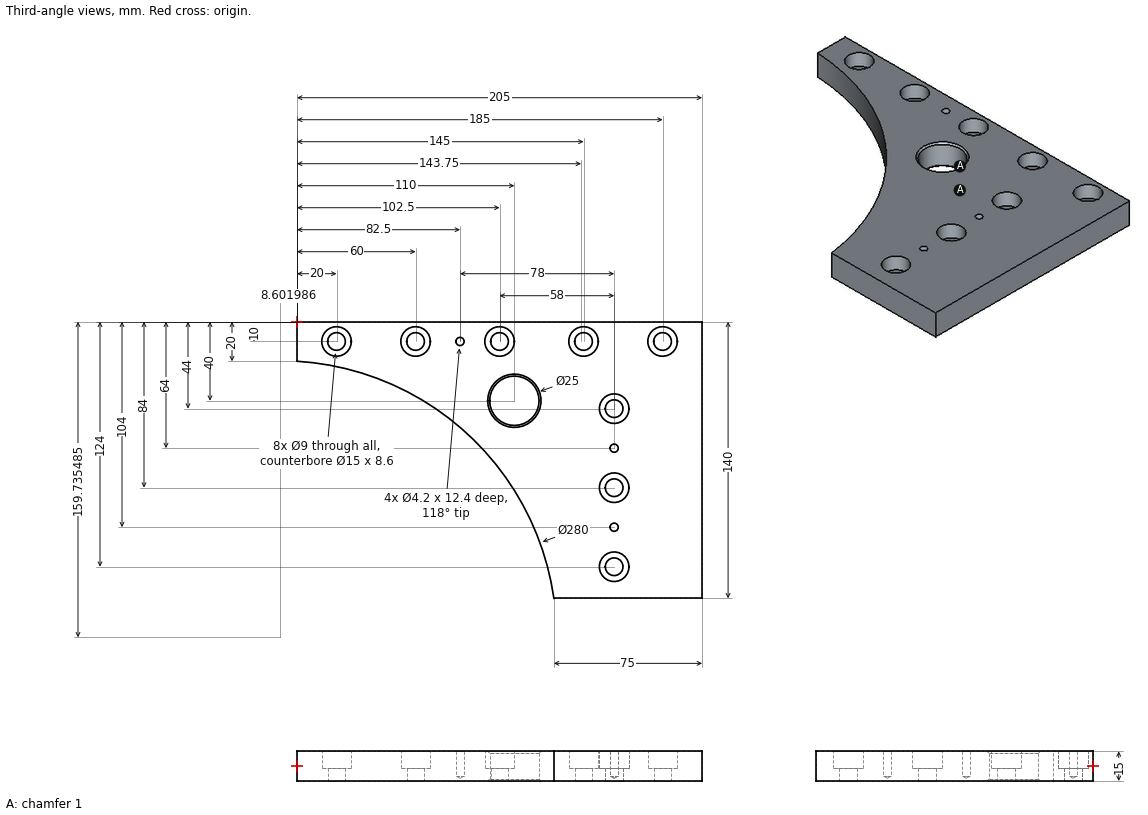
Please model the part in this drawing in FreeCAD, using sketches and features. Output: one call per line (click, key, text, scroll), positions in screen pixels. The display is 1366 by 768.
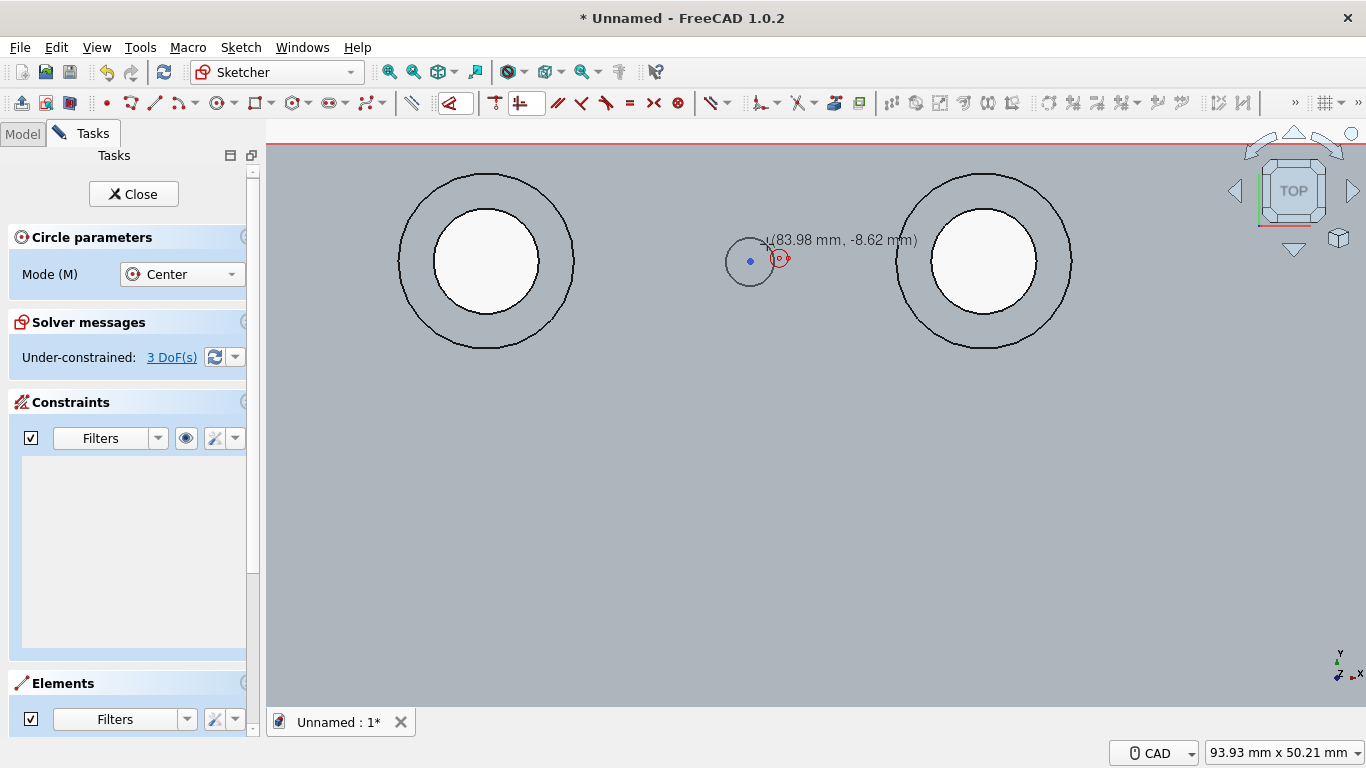
scroll(753, 261, down, 6)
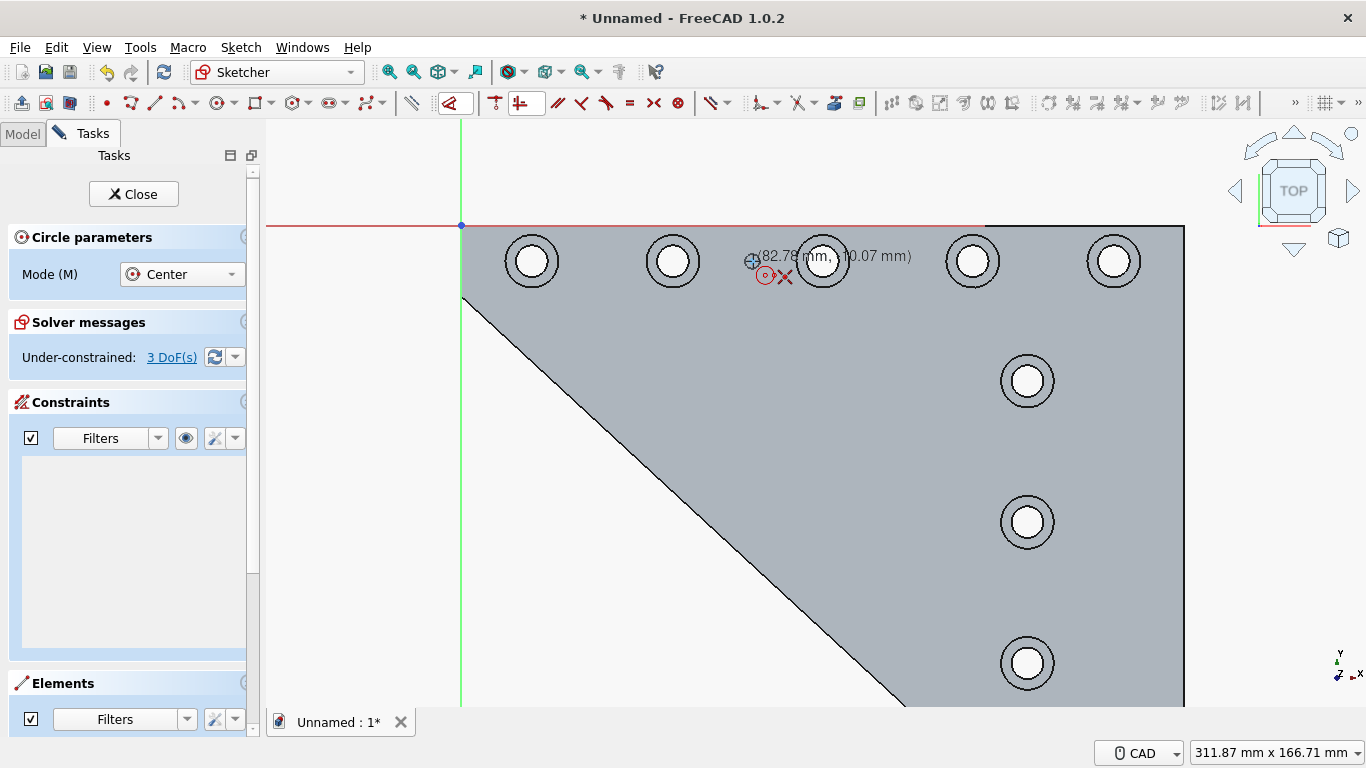
scroll(968, 261, up, 6)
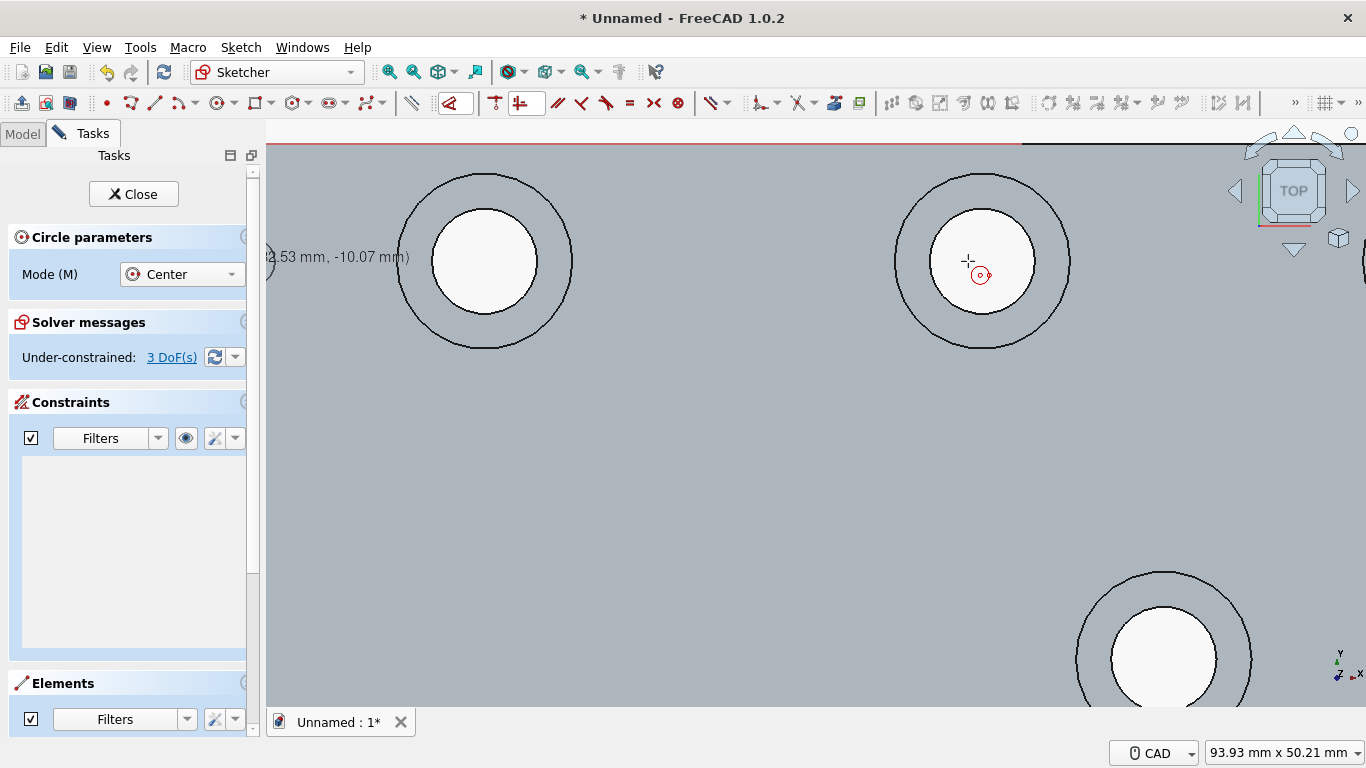
click(968, 261)
click(985, 244)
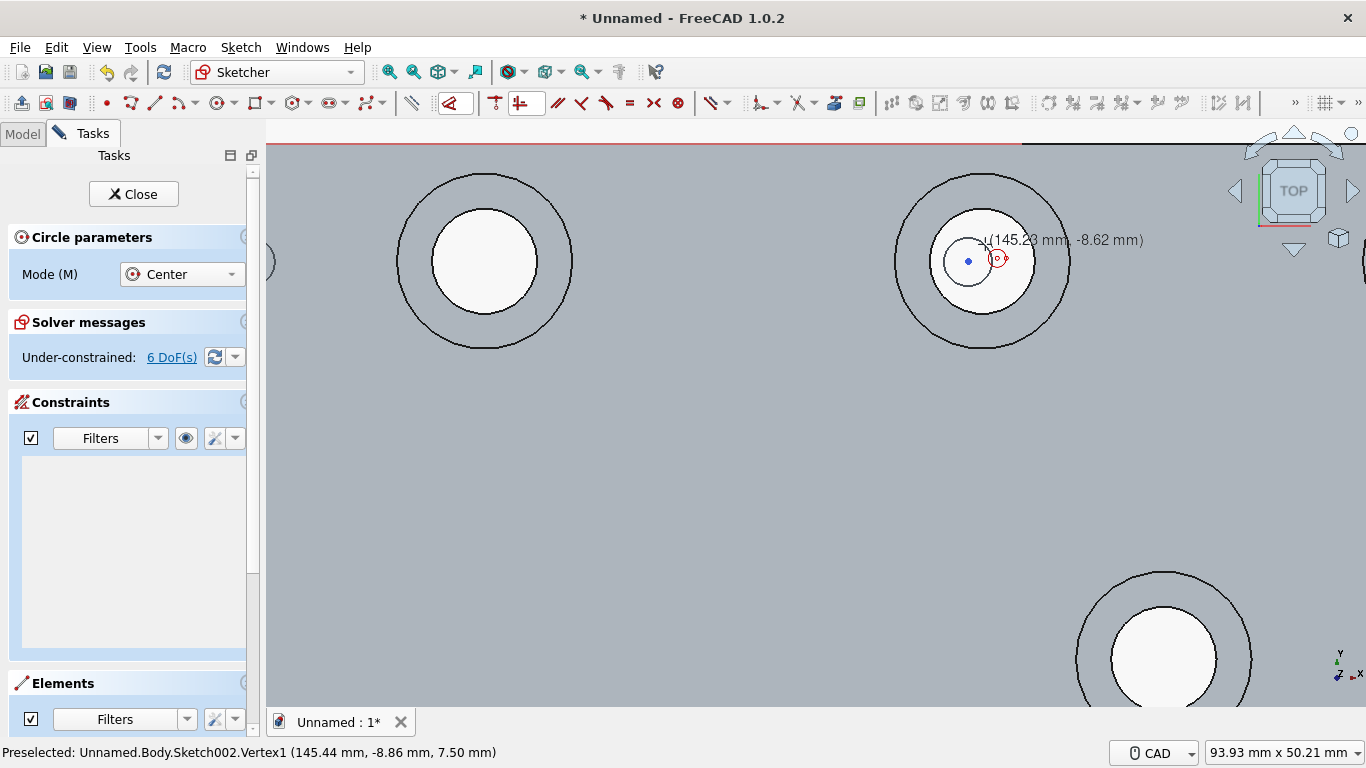
scroll(968, 261, down, 6)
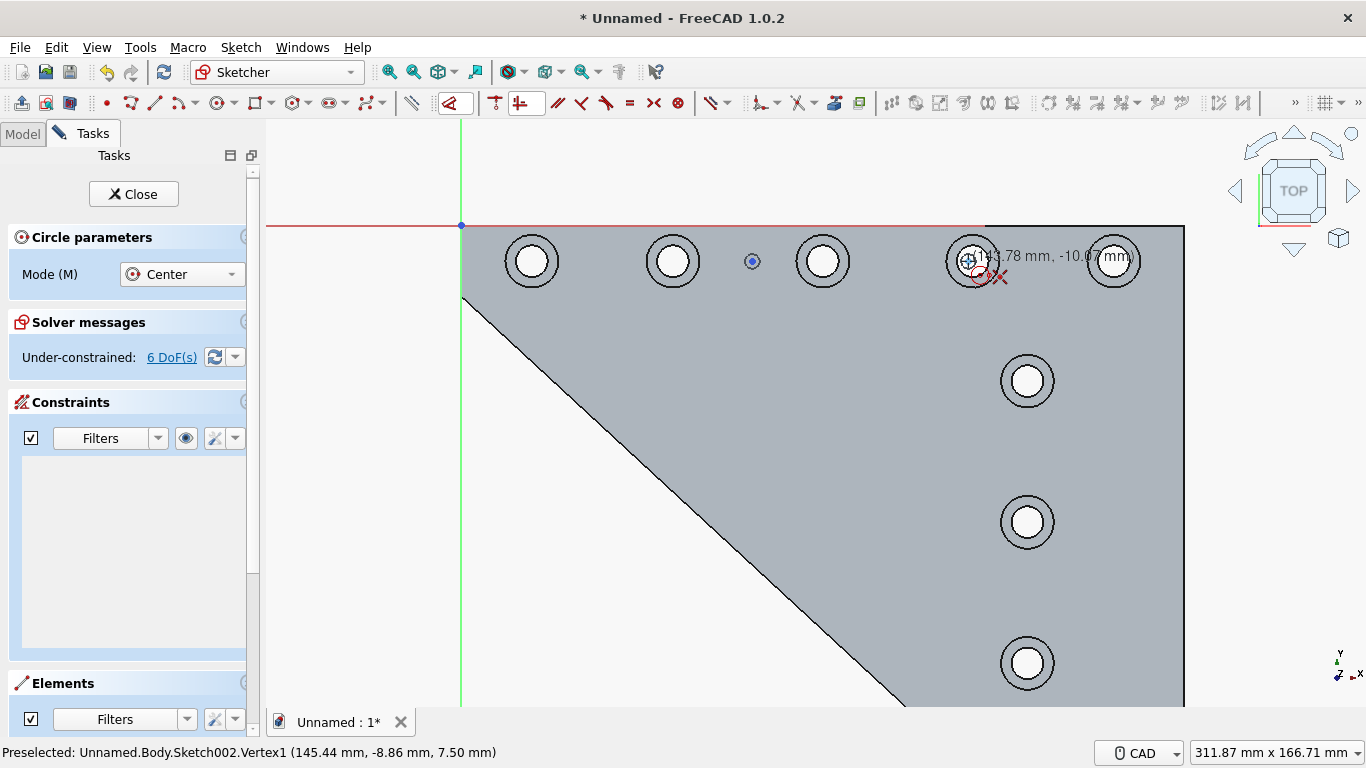
scroll(1027, 452, up, 6)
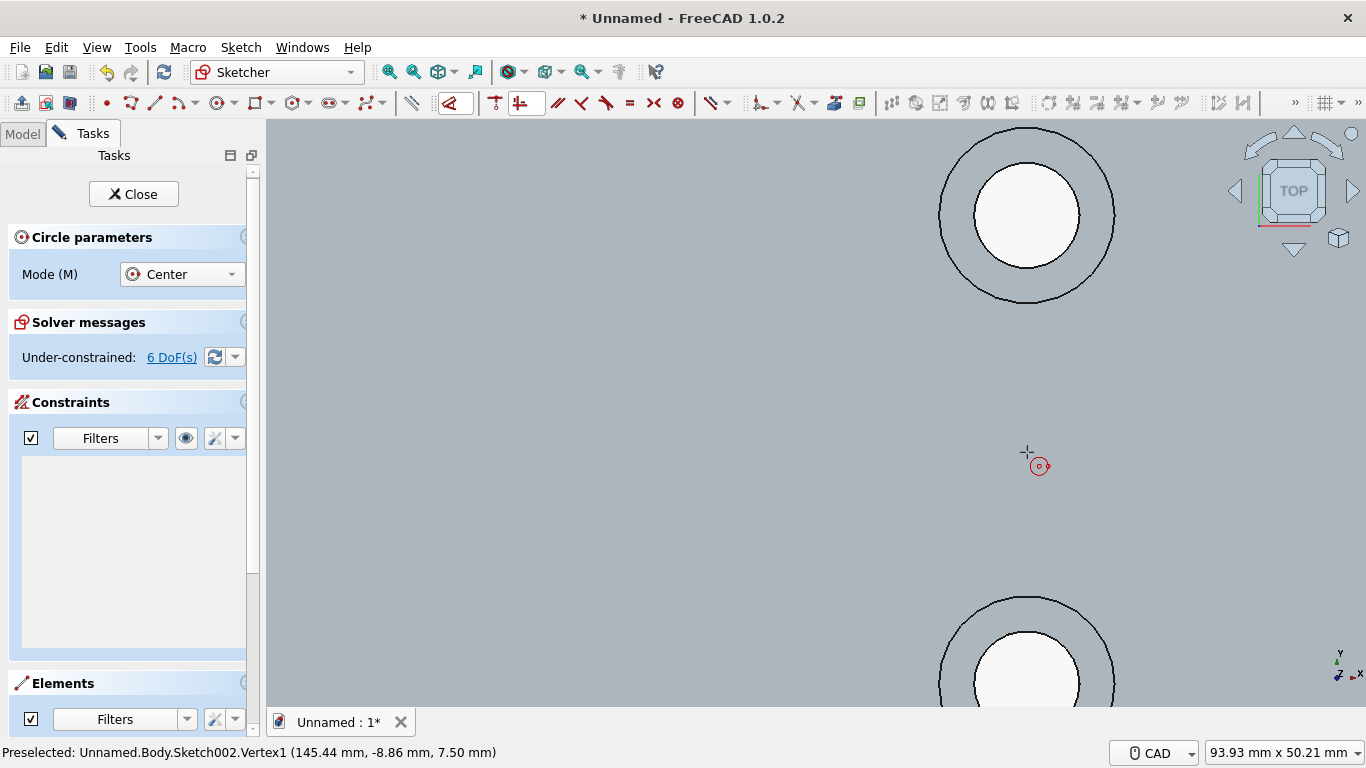
click(1027, 450)
click(1044, 432)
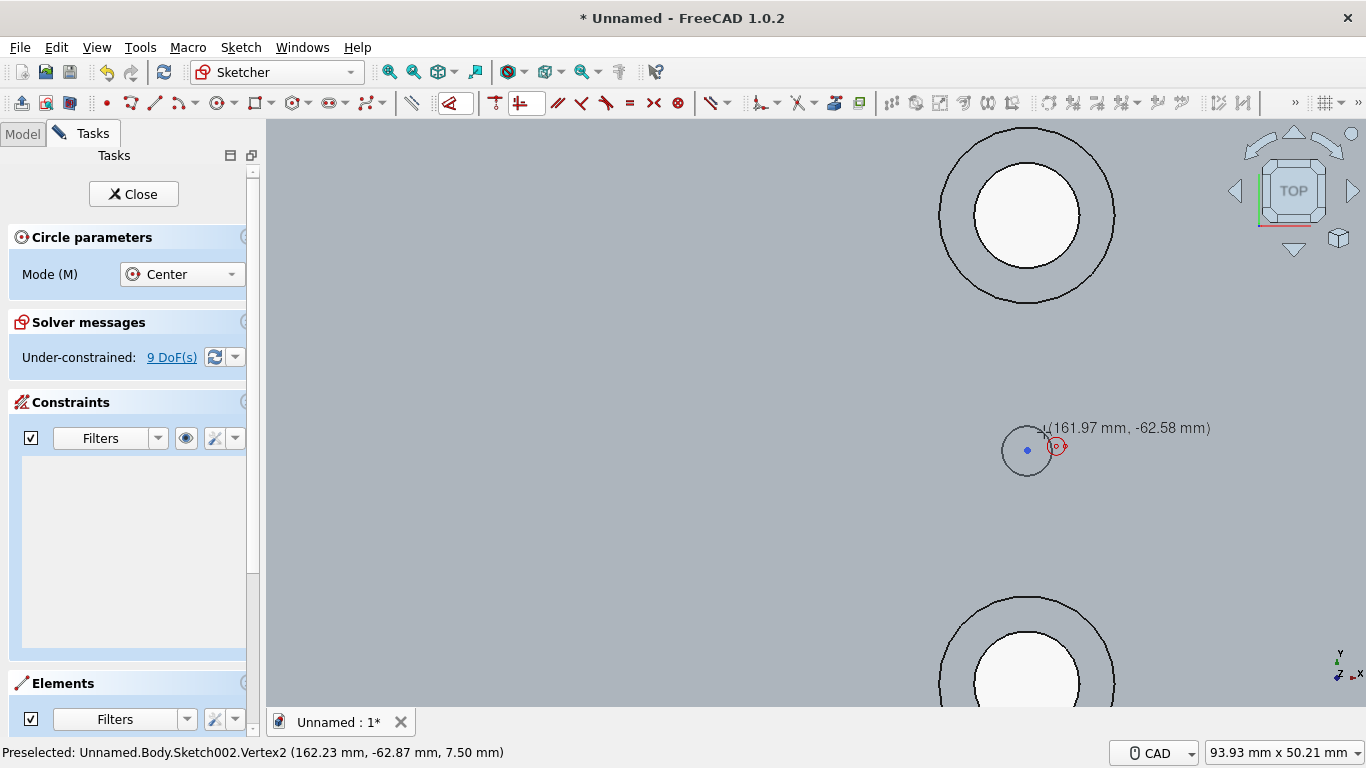
scroll(1027, 452, down, 6)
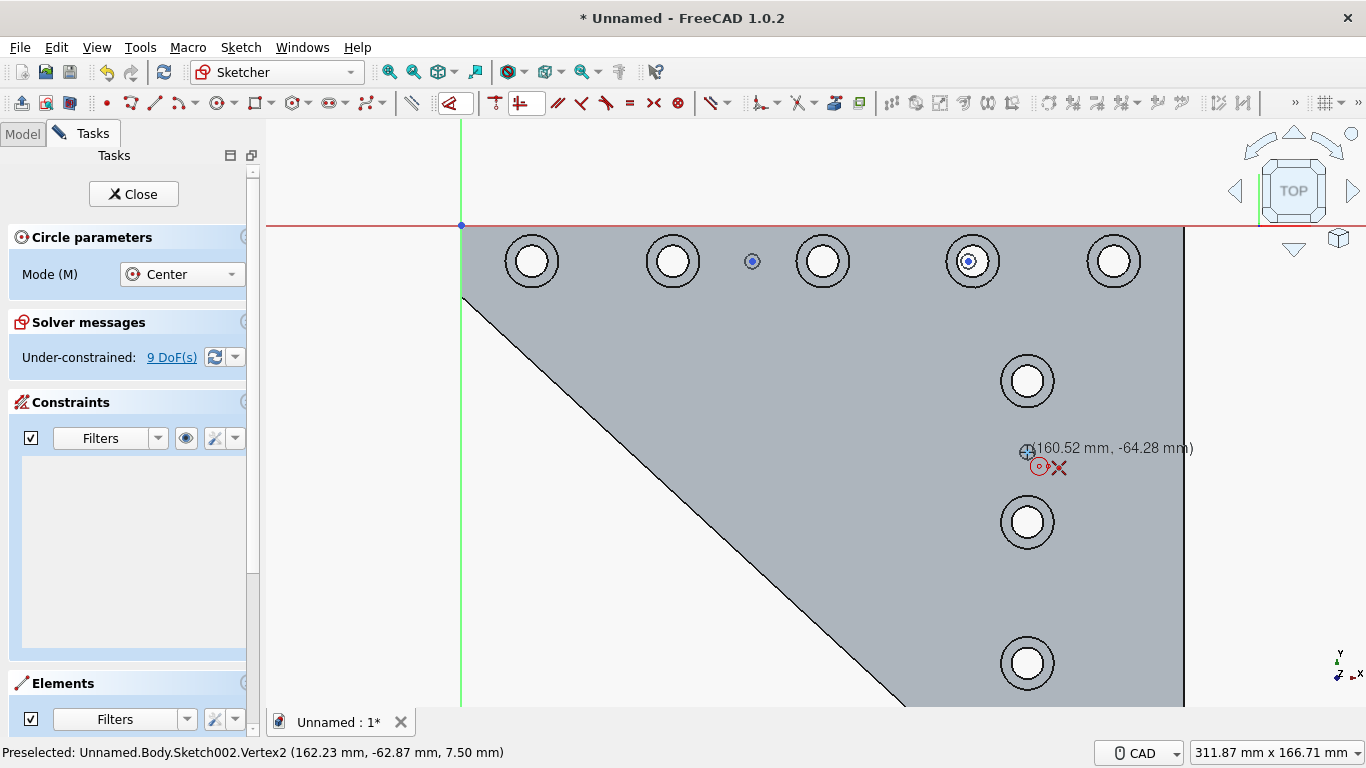
scroll(1027, 593, up, 6)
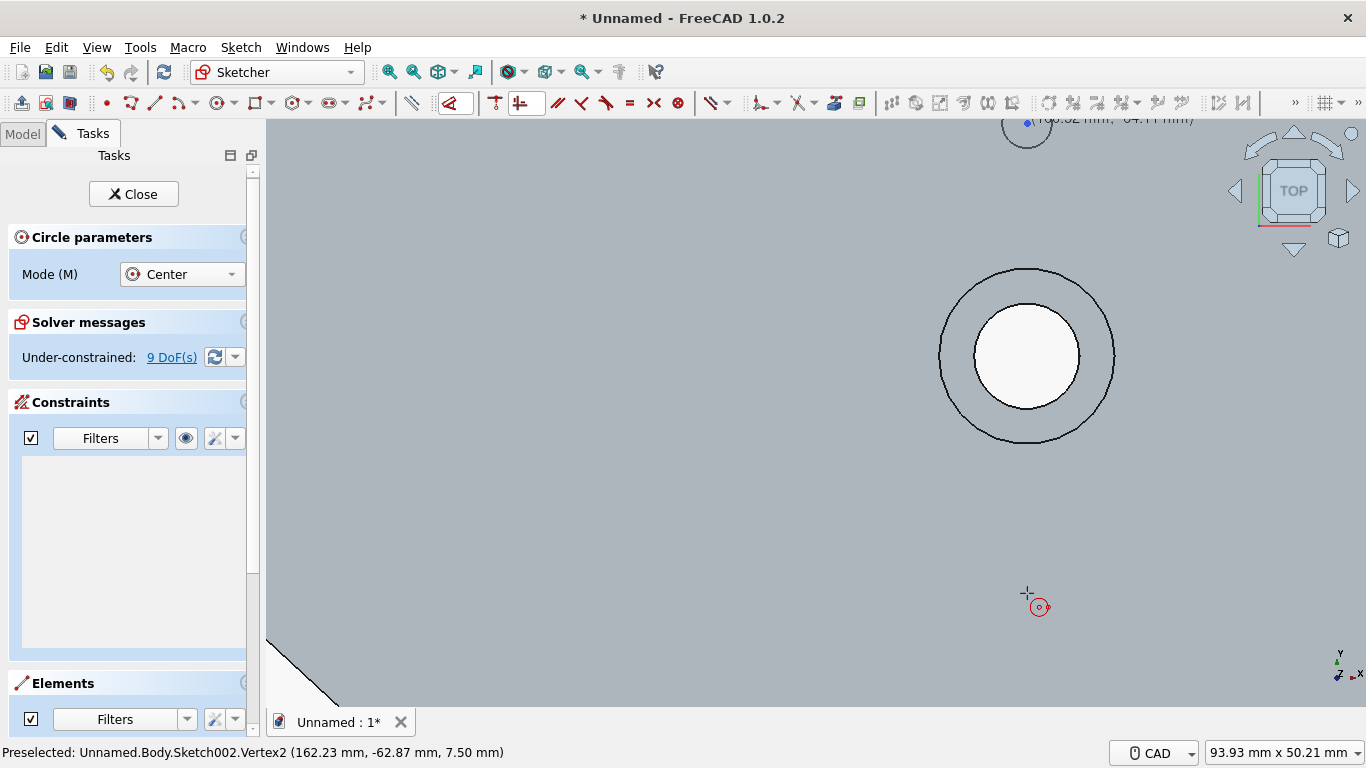
click(1027, 590)
click(1044, 573)
key(Escape)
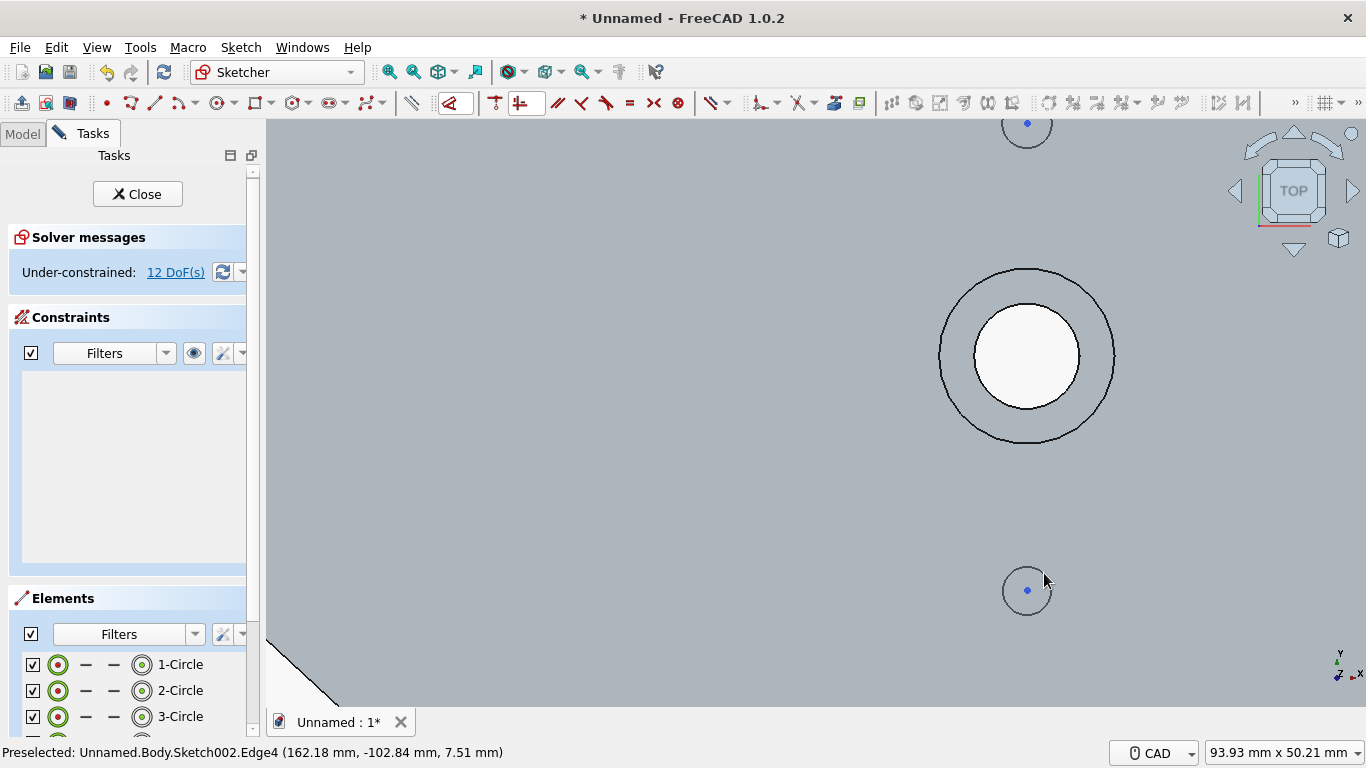
scroll(1027, 594, down, 6)